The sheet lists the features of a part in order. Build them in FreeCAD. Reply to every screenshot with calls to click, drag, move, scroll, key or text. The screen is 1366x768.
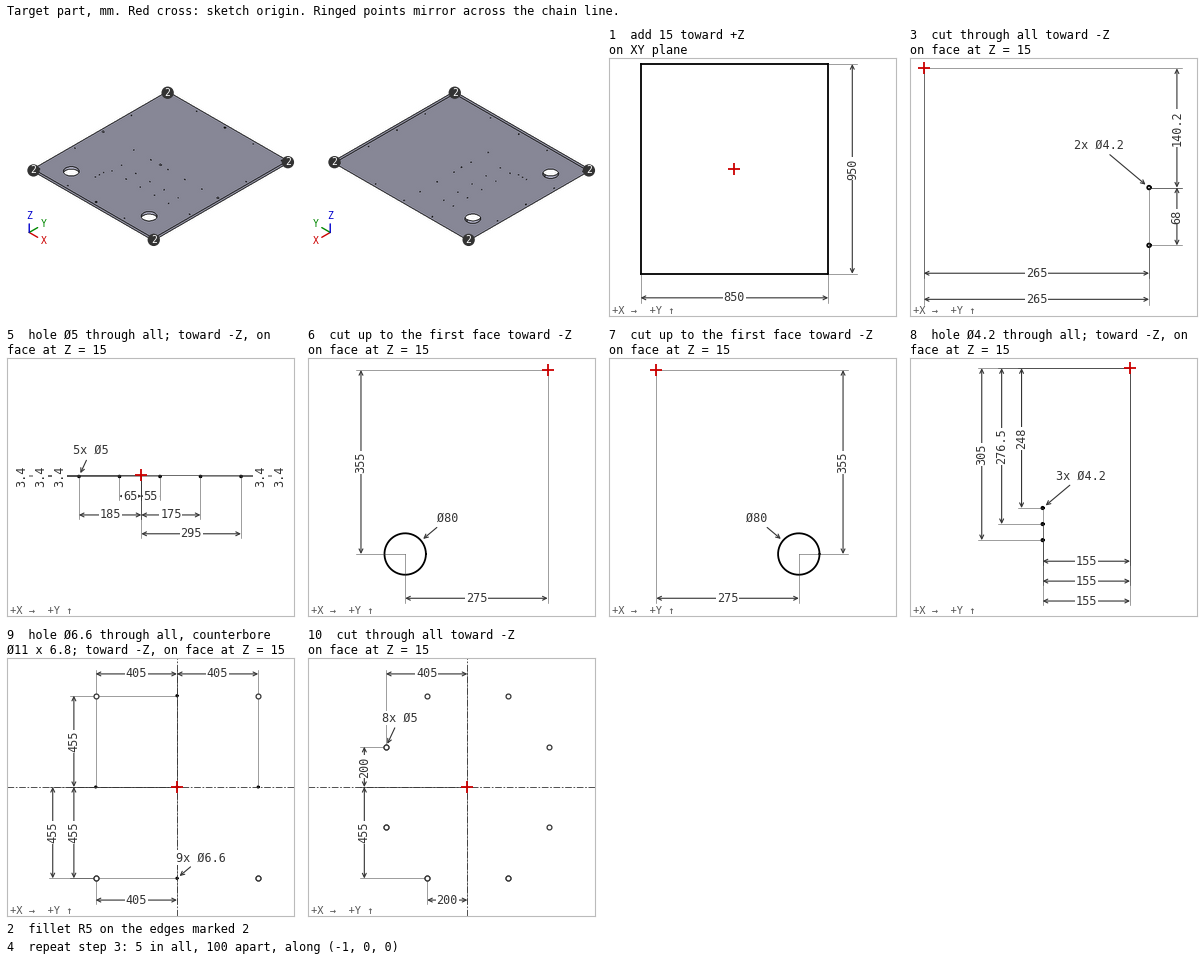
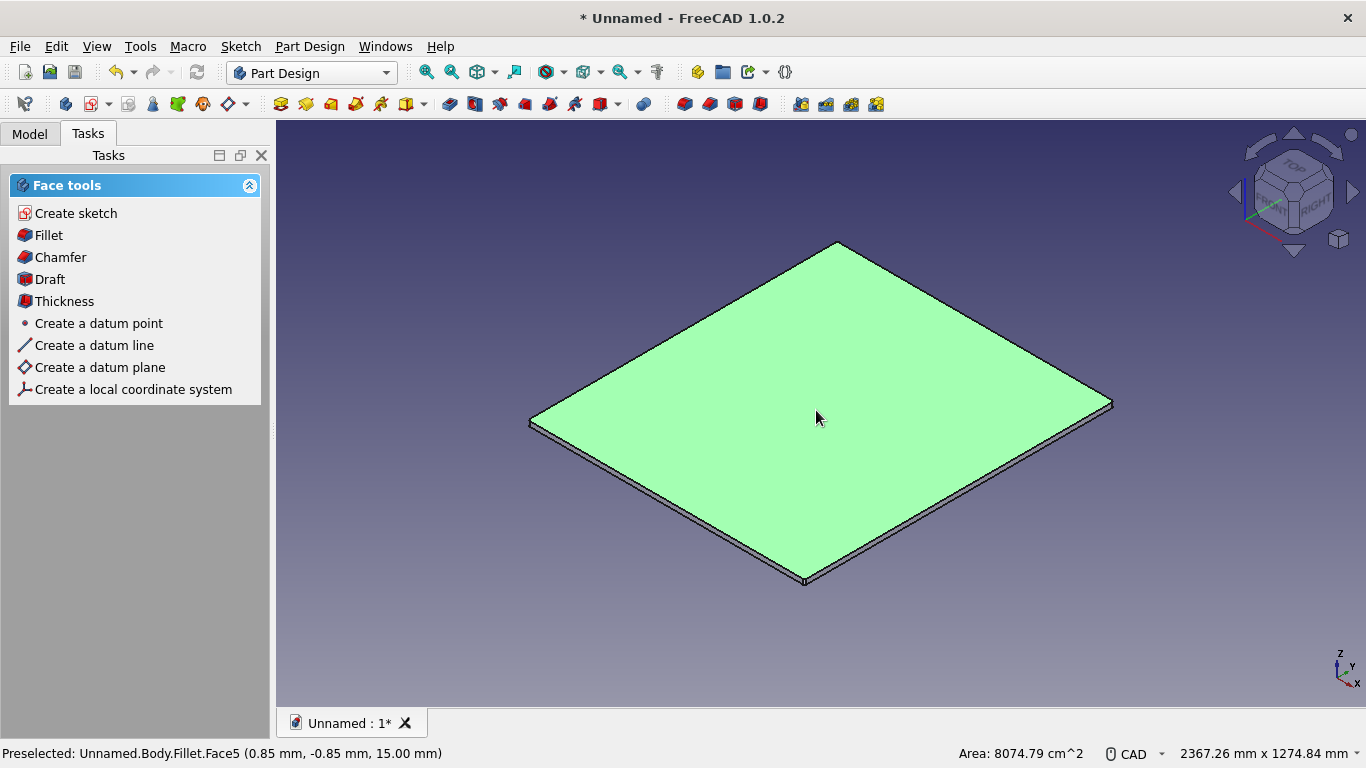
click(90, 104)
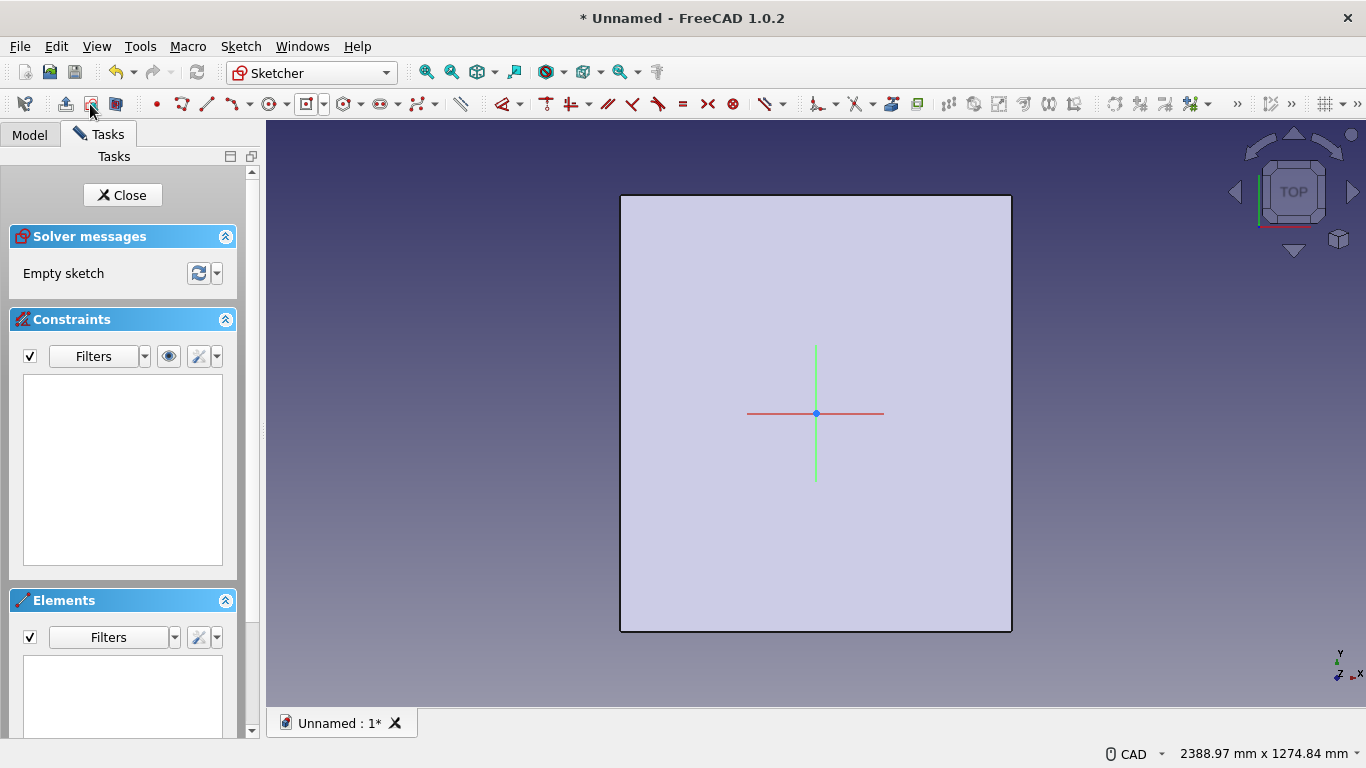
scroll(957, 502, up, 12)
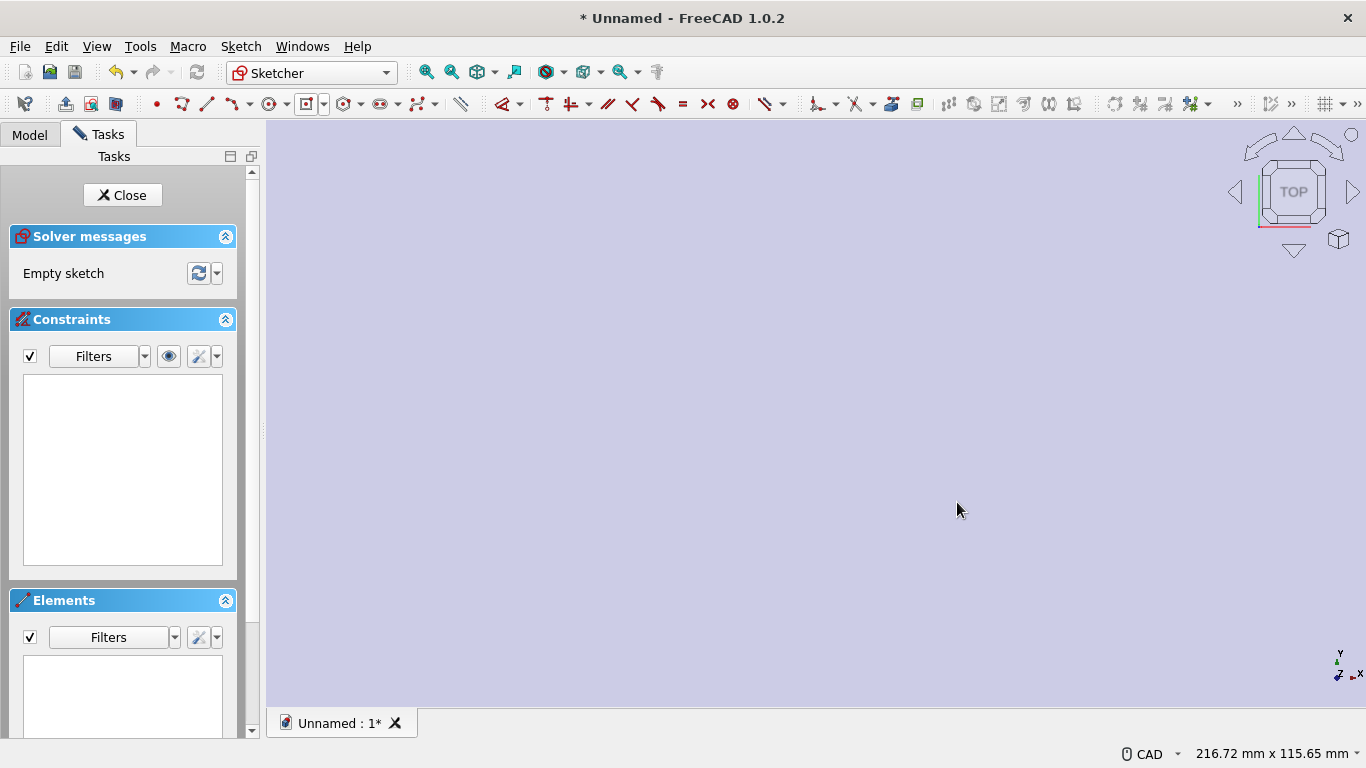
click(268, 104)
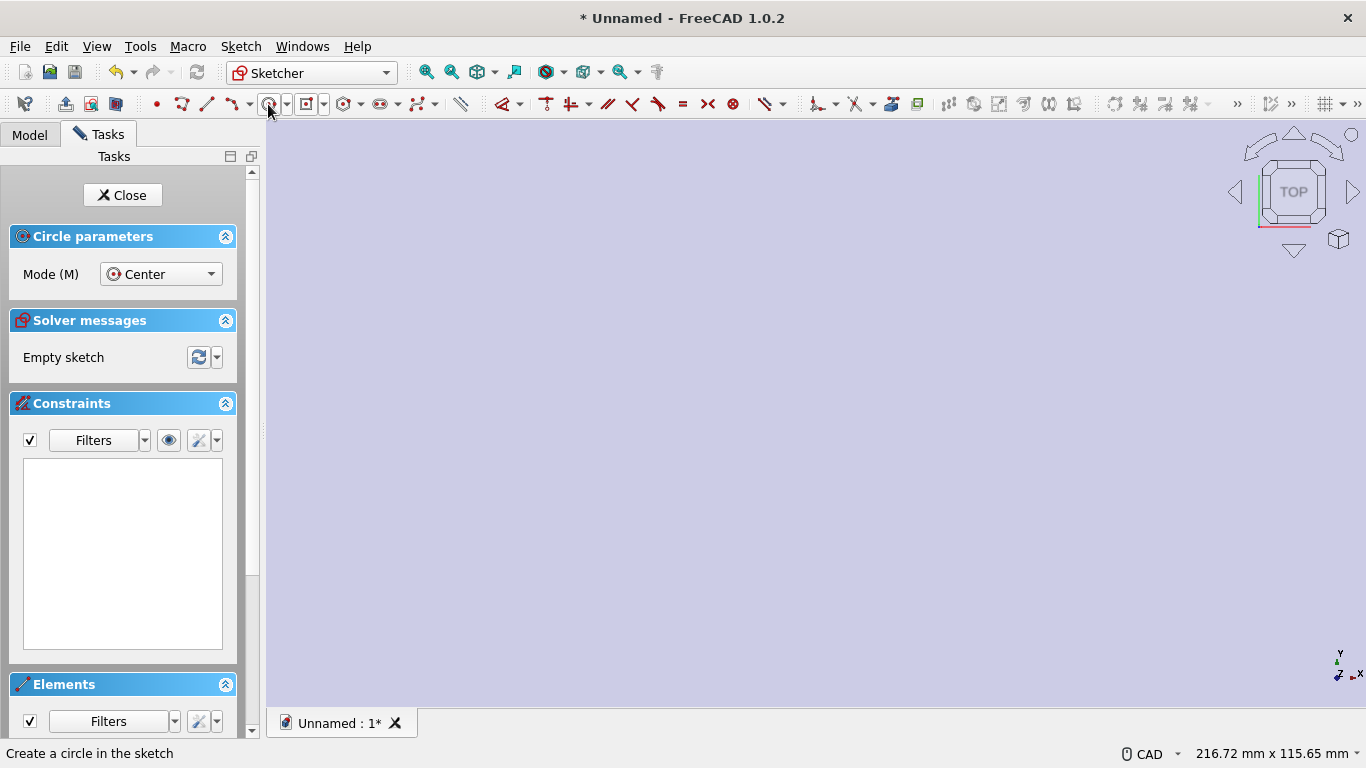
scroll(741, 232, up, 4)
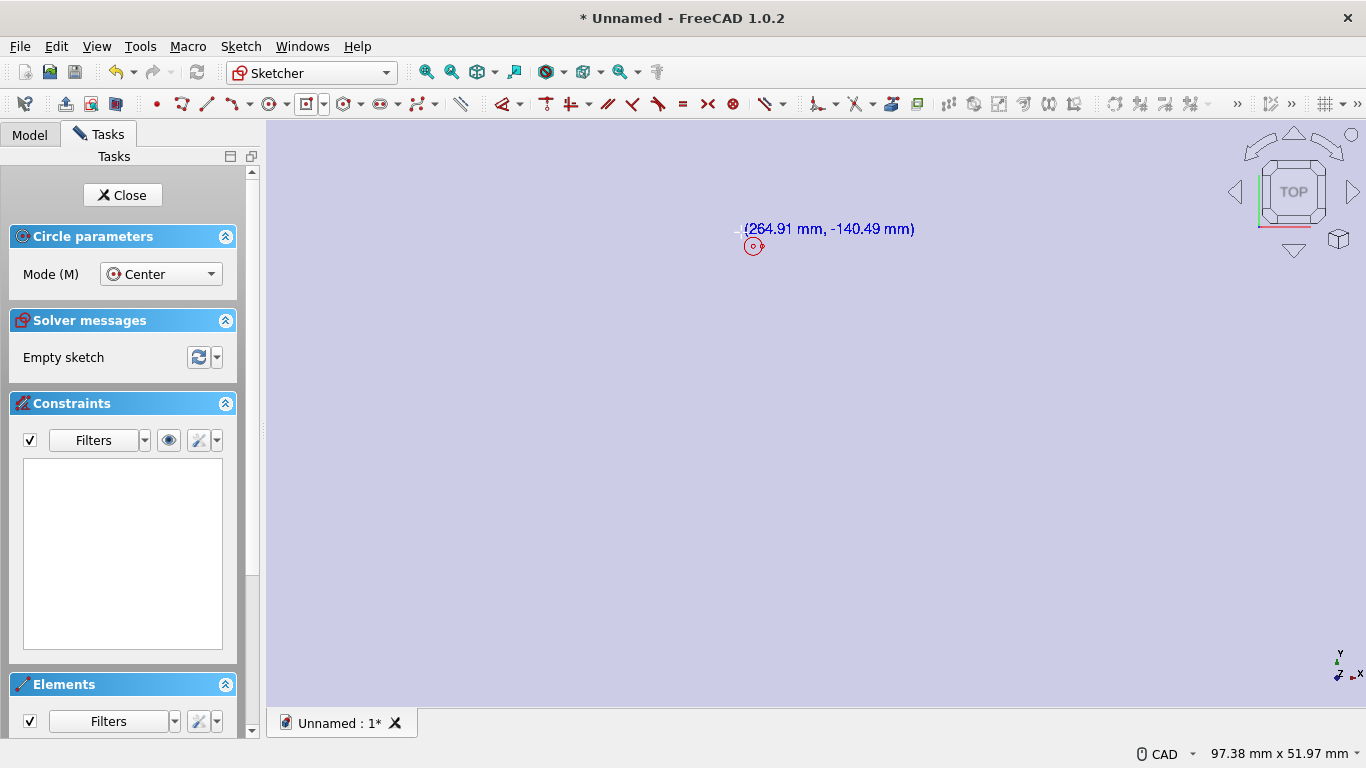
click(742, 231)
move(758, 214)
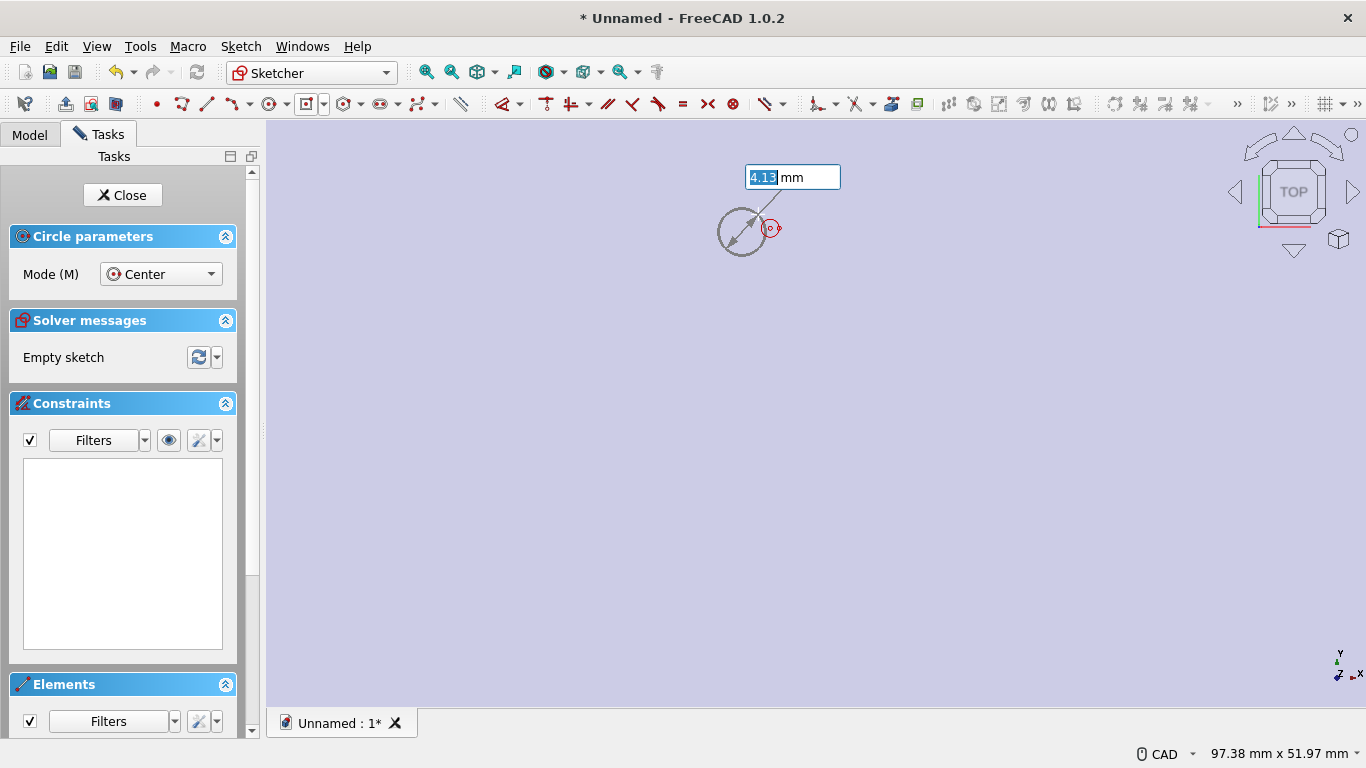
text(4.2)
key(Return)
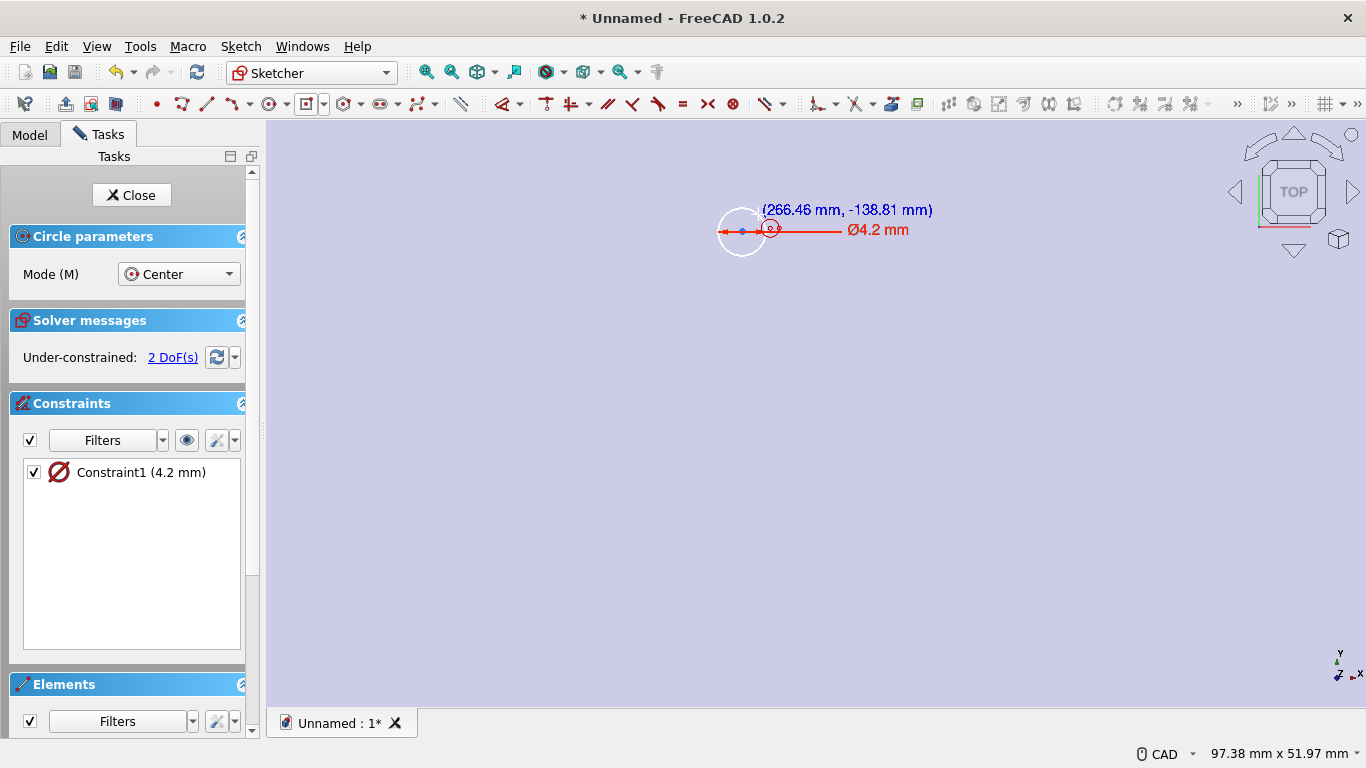
scroll(752, 249, down, 4)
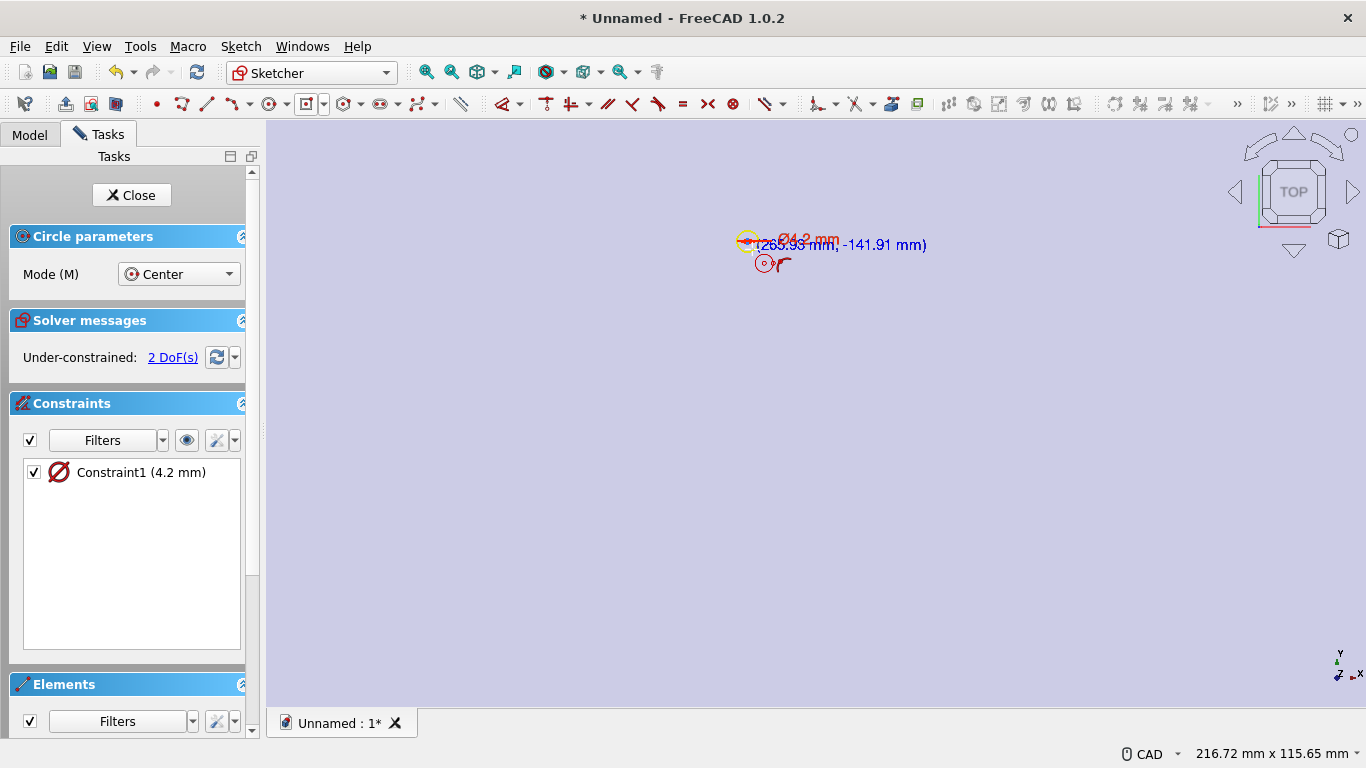
scroll(748, 586, up, 4)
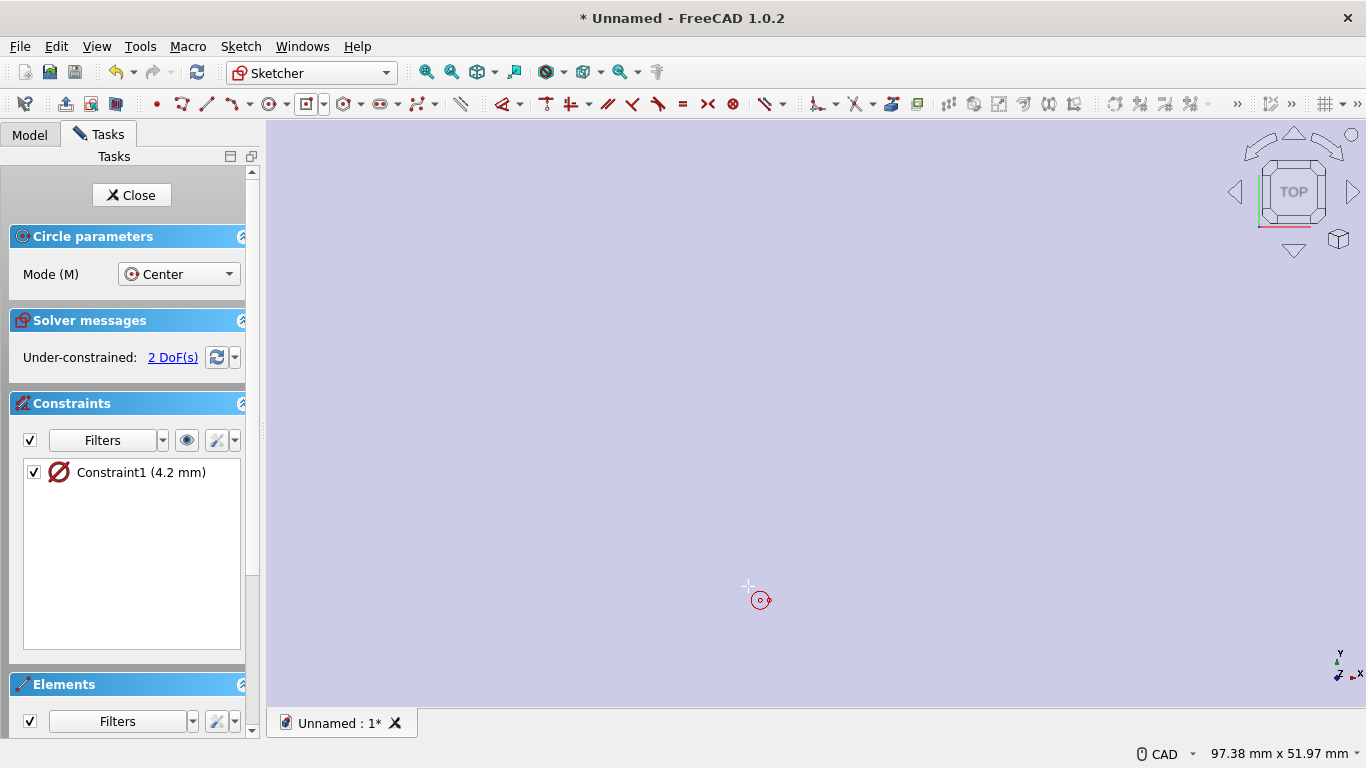
click(746, 585)
move(763, 568)